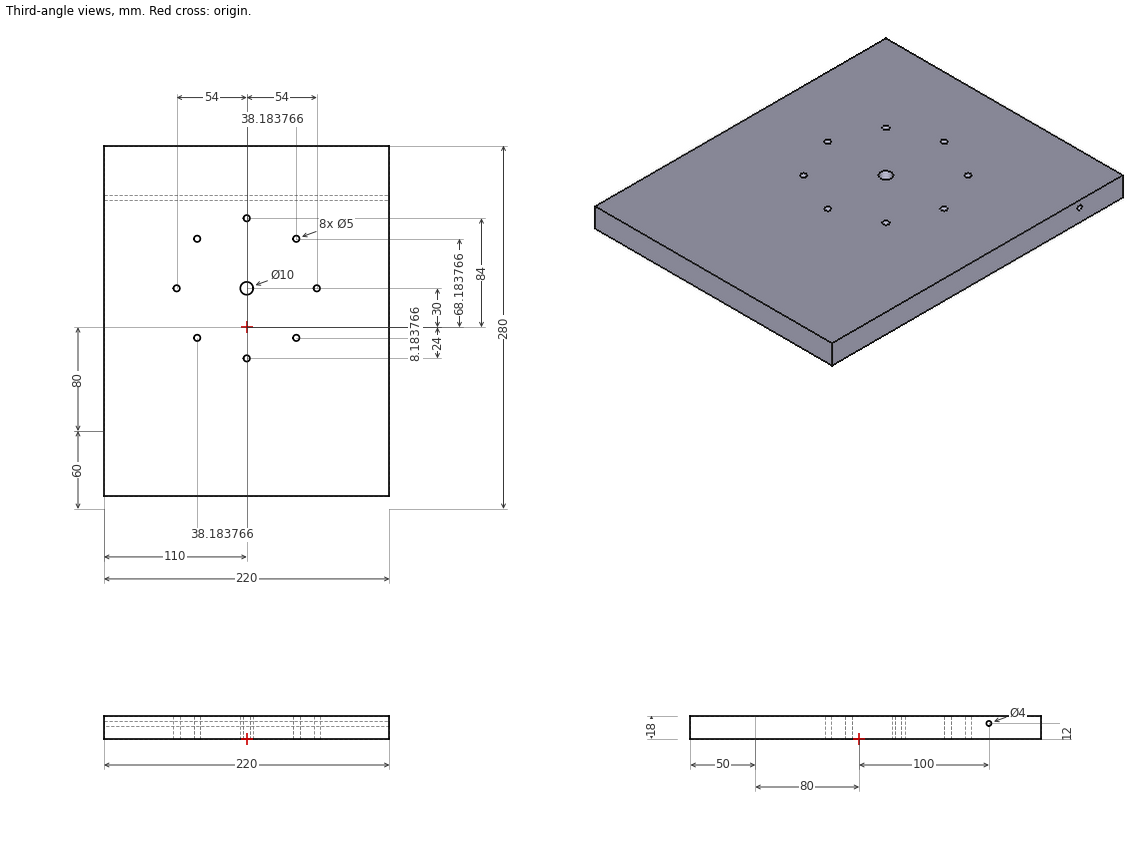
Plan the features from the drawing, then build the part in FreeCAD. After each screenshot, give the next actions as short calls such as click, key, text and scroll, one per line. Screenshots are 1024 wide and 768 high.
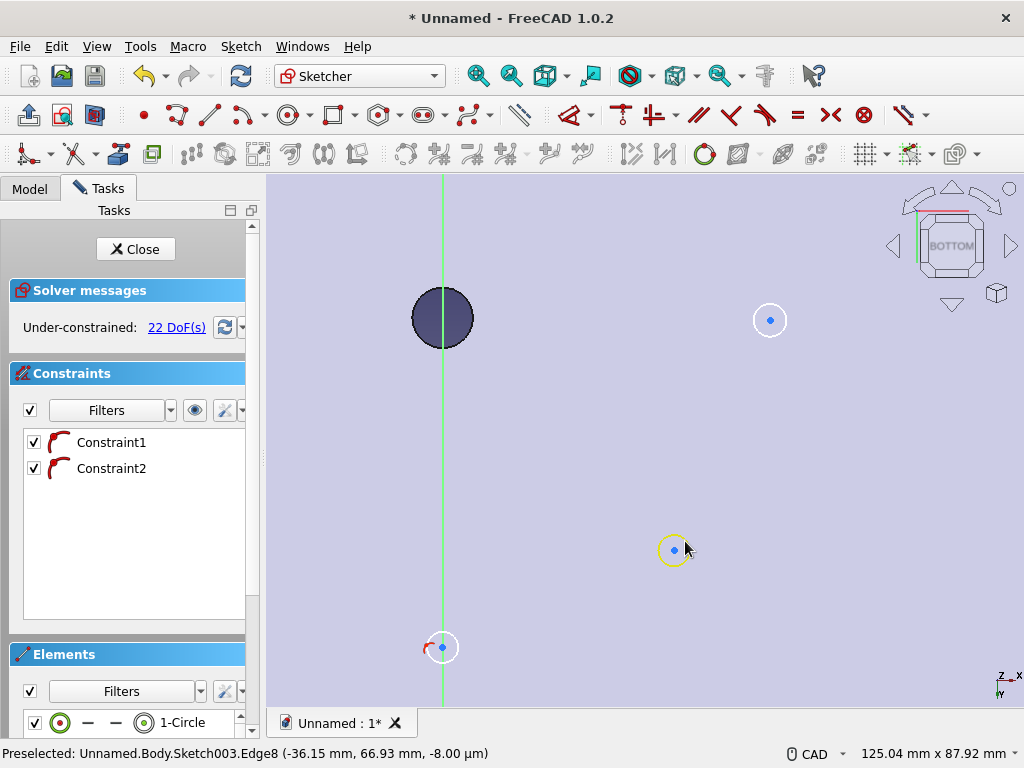
click(685, 540)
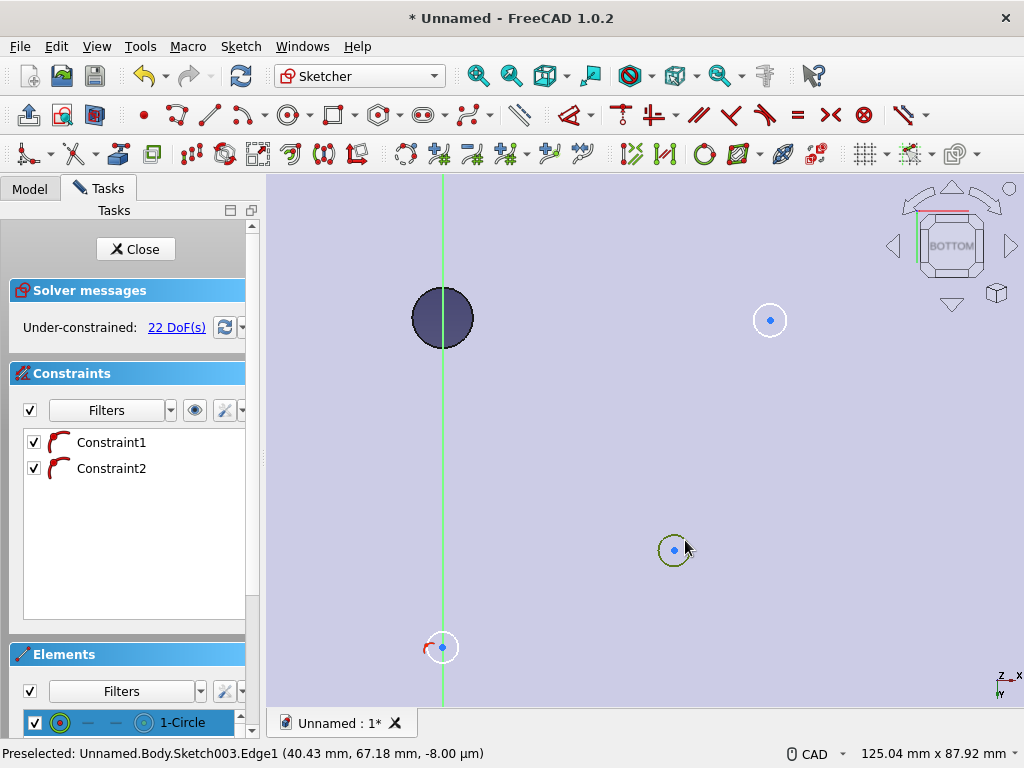
scroll(454, 636, up, 2)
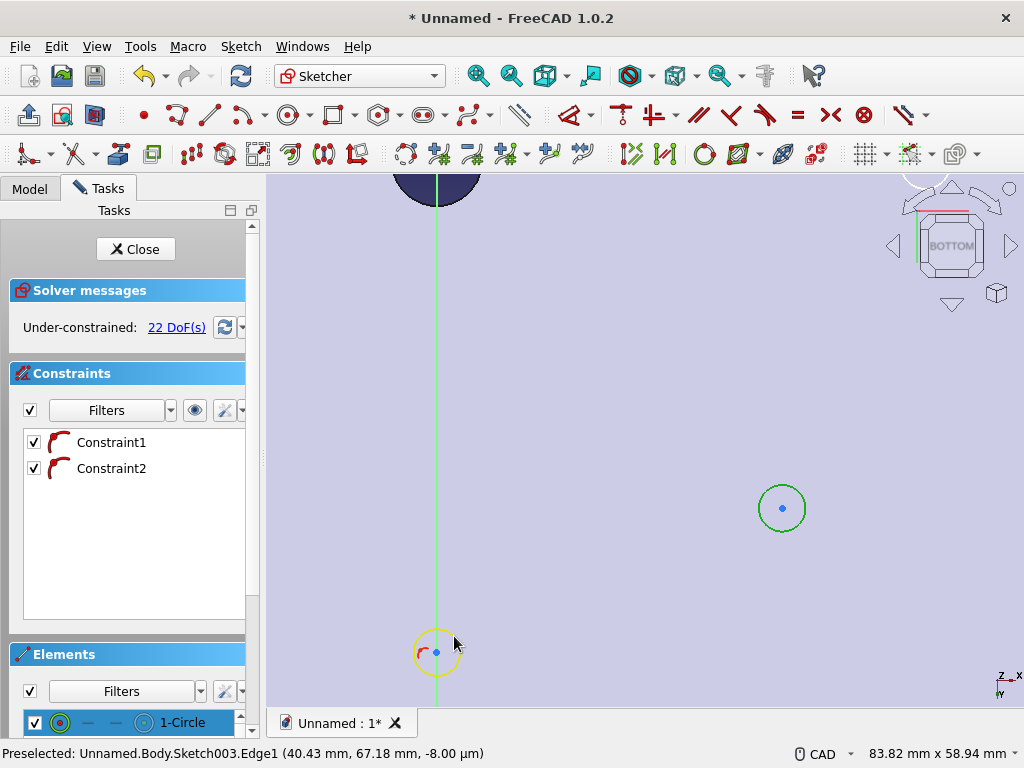
click(453, 636)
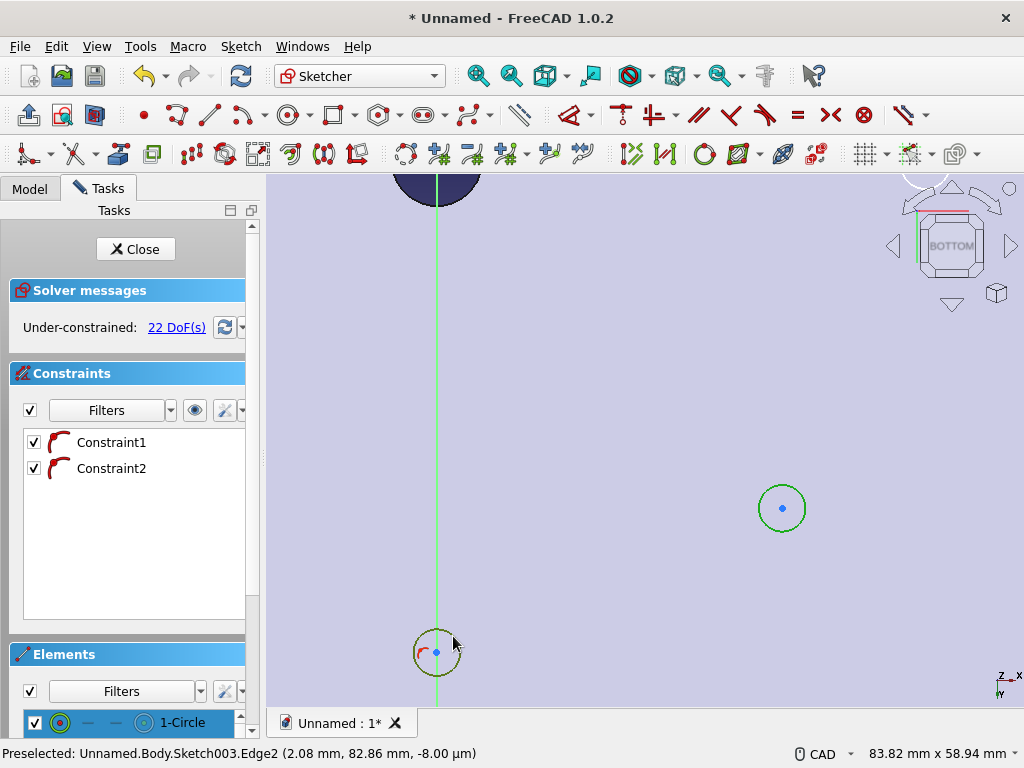
scroll(637, 561, down, 6)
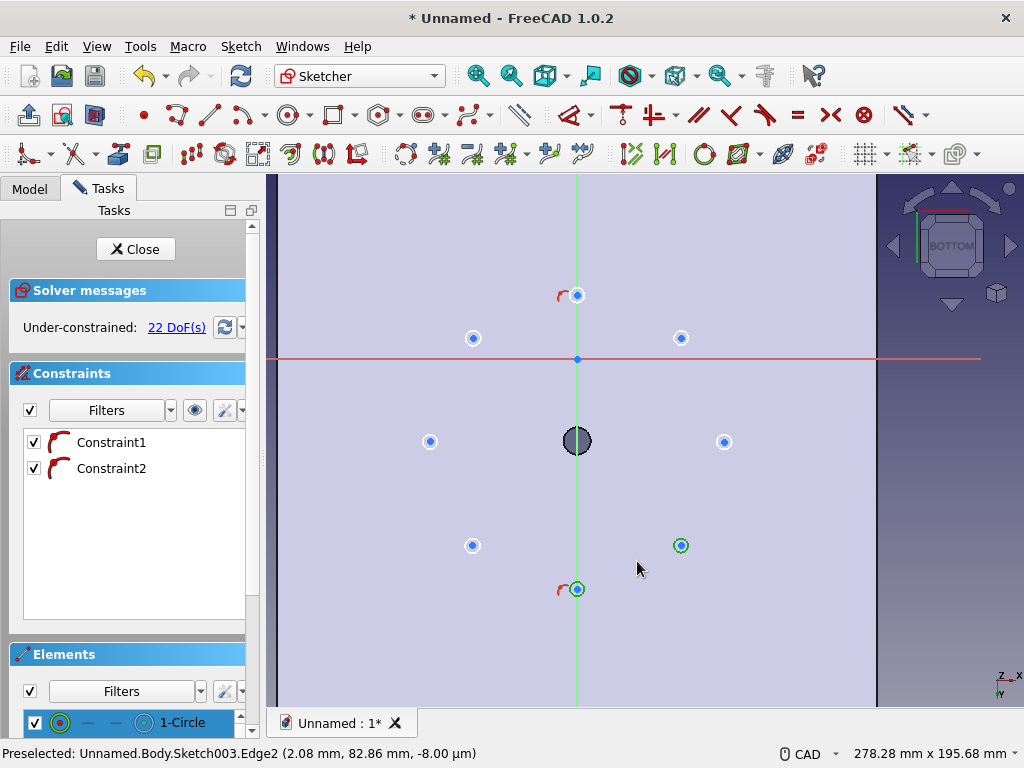
scroll(729, 437, up, 4)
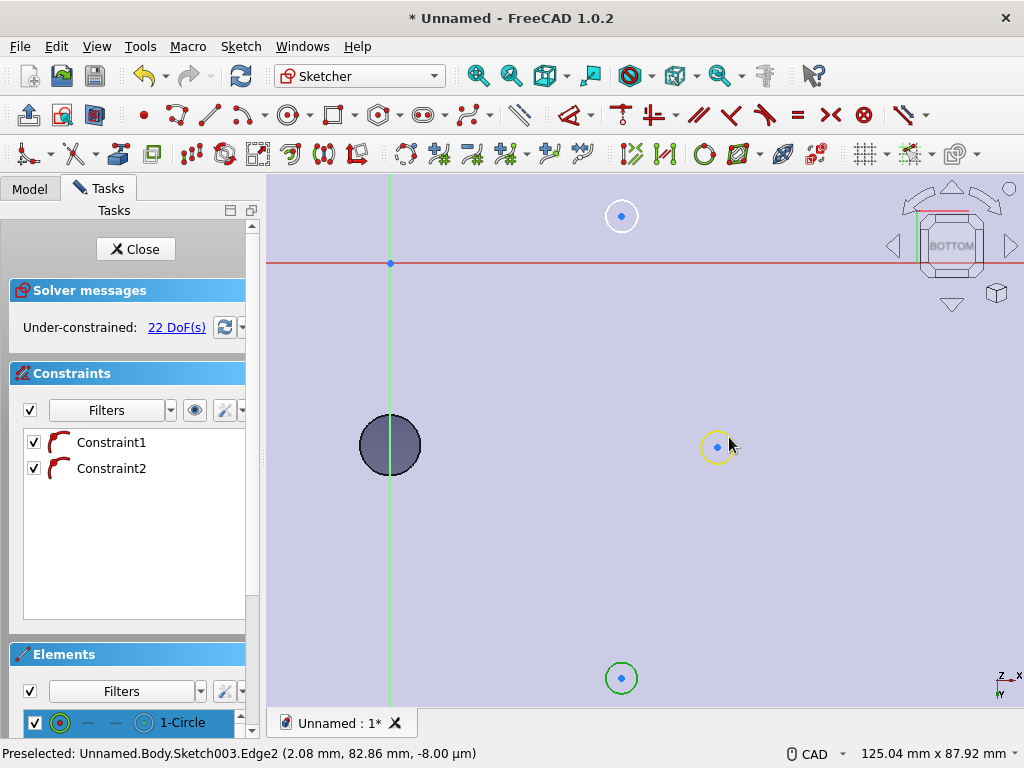
click(729, 436)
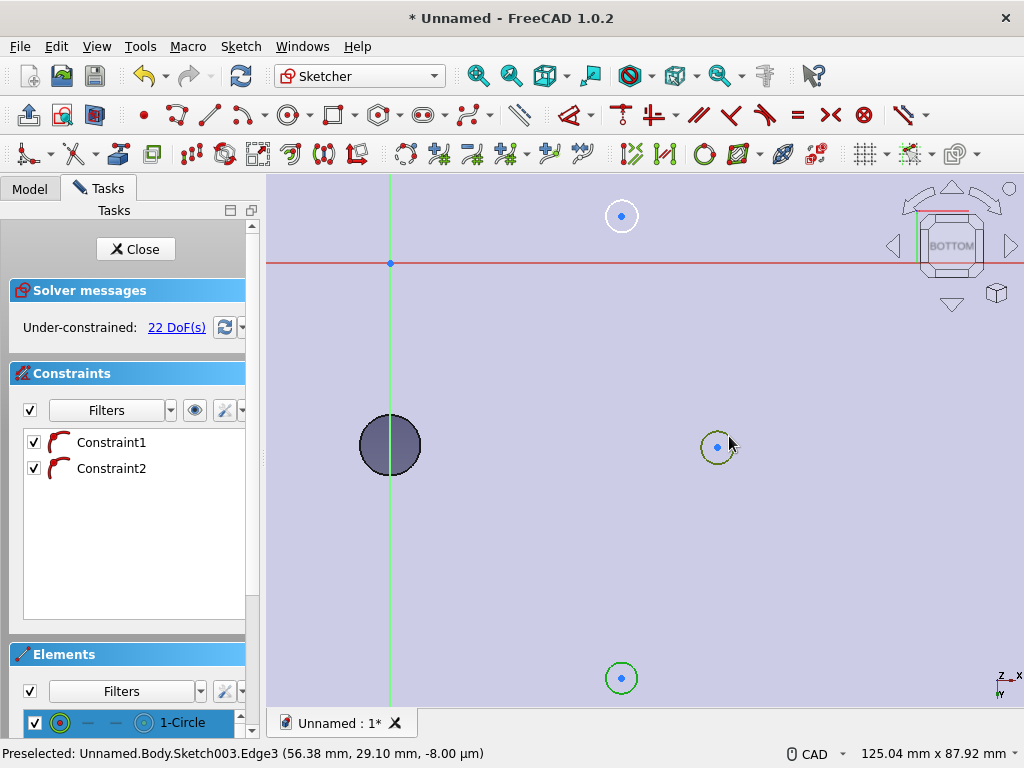
click(633, 205)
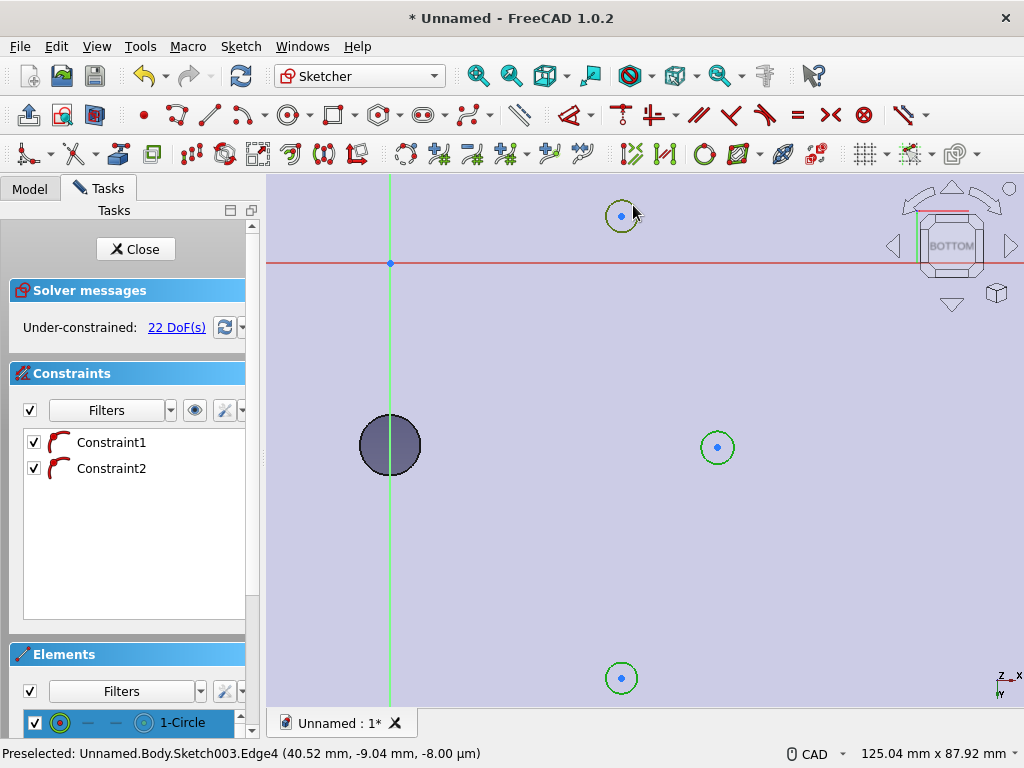
scroll(729, 437, down, 4)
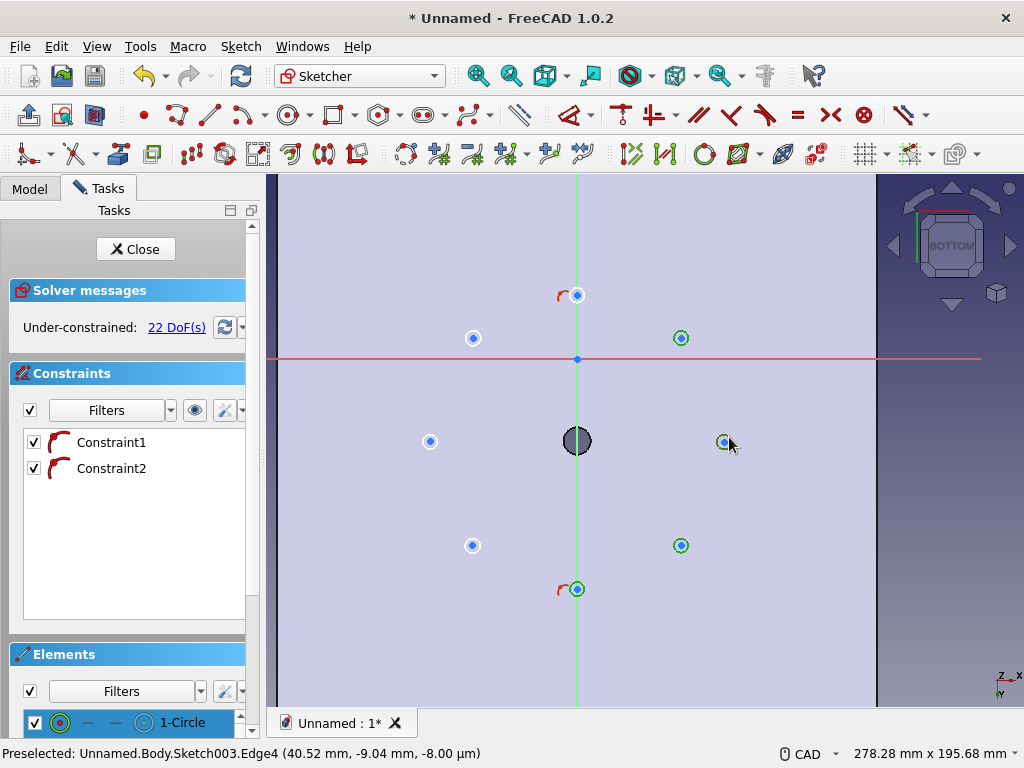
scroll(582, 290, up, 5)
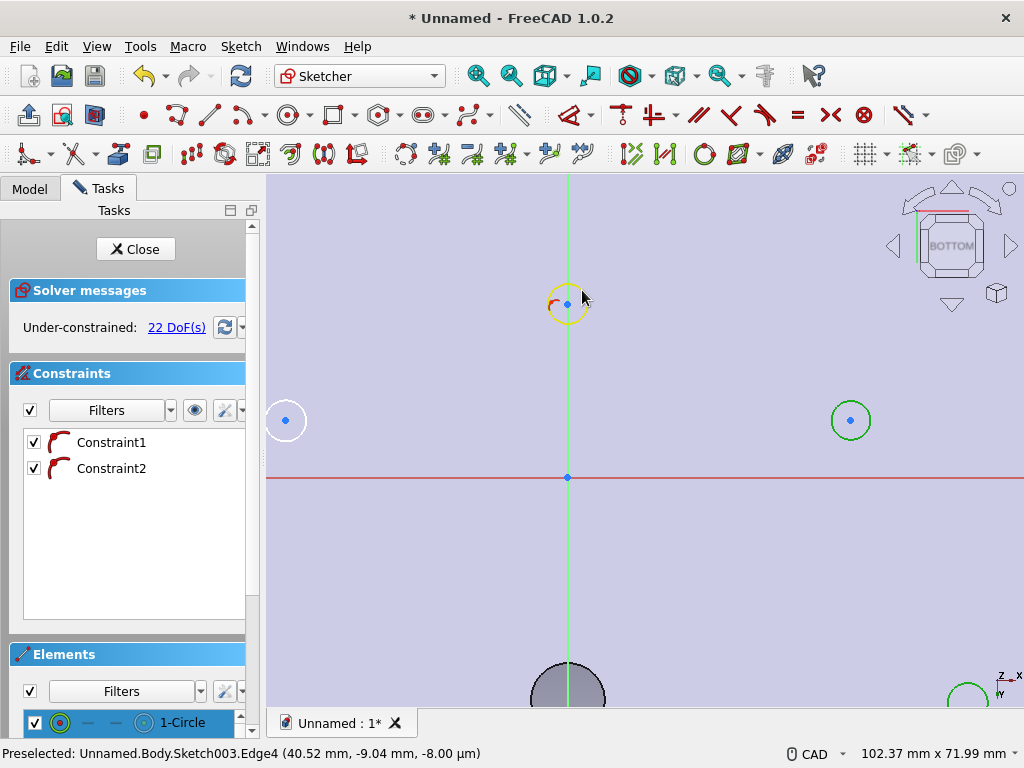
click(582, 290)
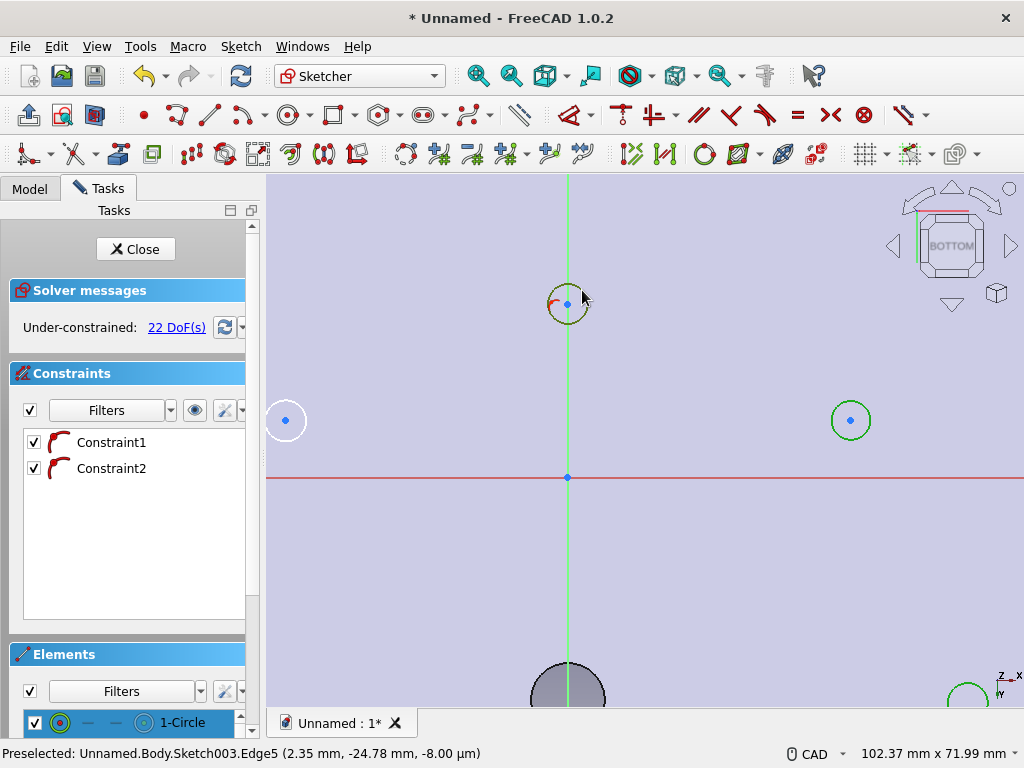
click(300, 406)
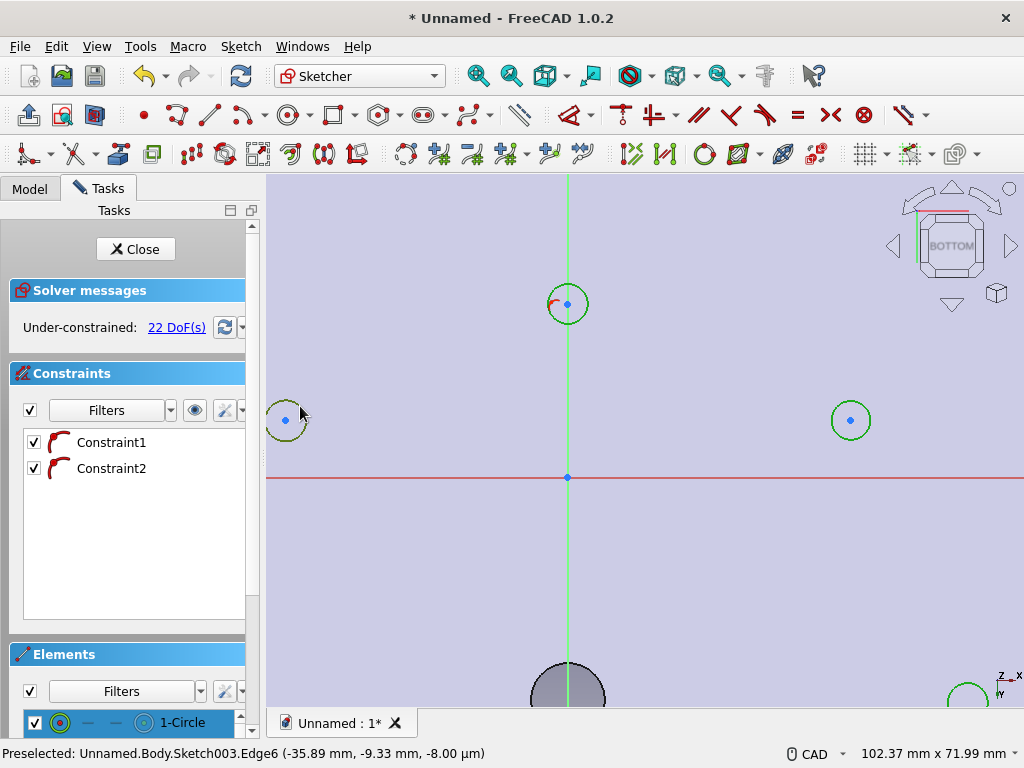
scroll(581, 289, down, 5)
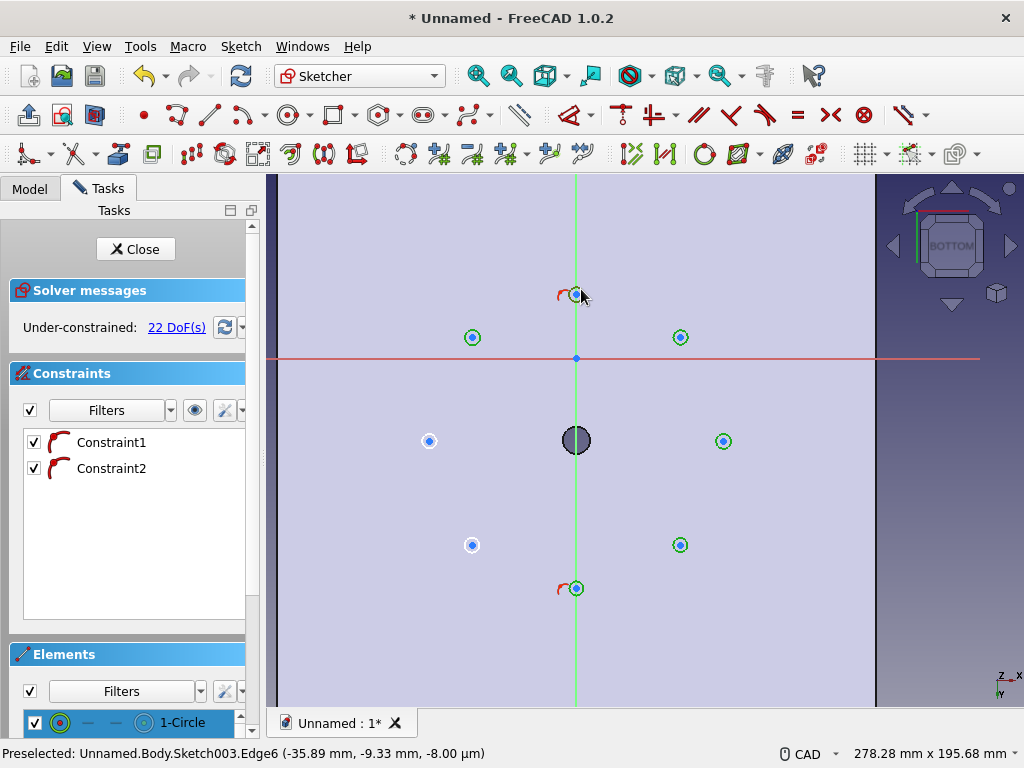
scroll(434, 436, up, 4)